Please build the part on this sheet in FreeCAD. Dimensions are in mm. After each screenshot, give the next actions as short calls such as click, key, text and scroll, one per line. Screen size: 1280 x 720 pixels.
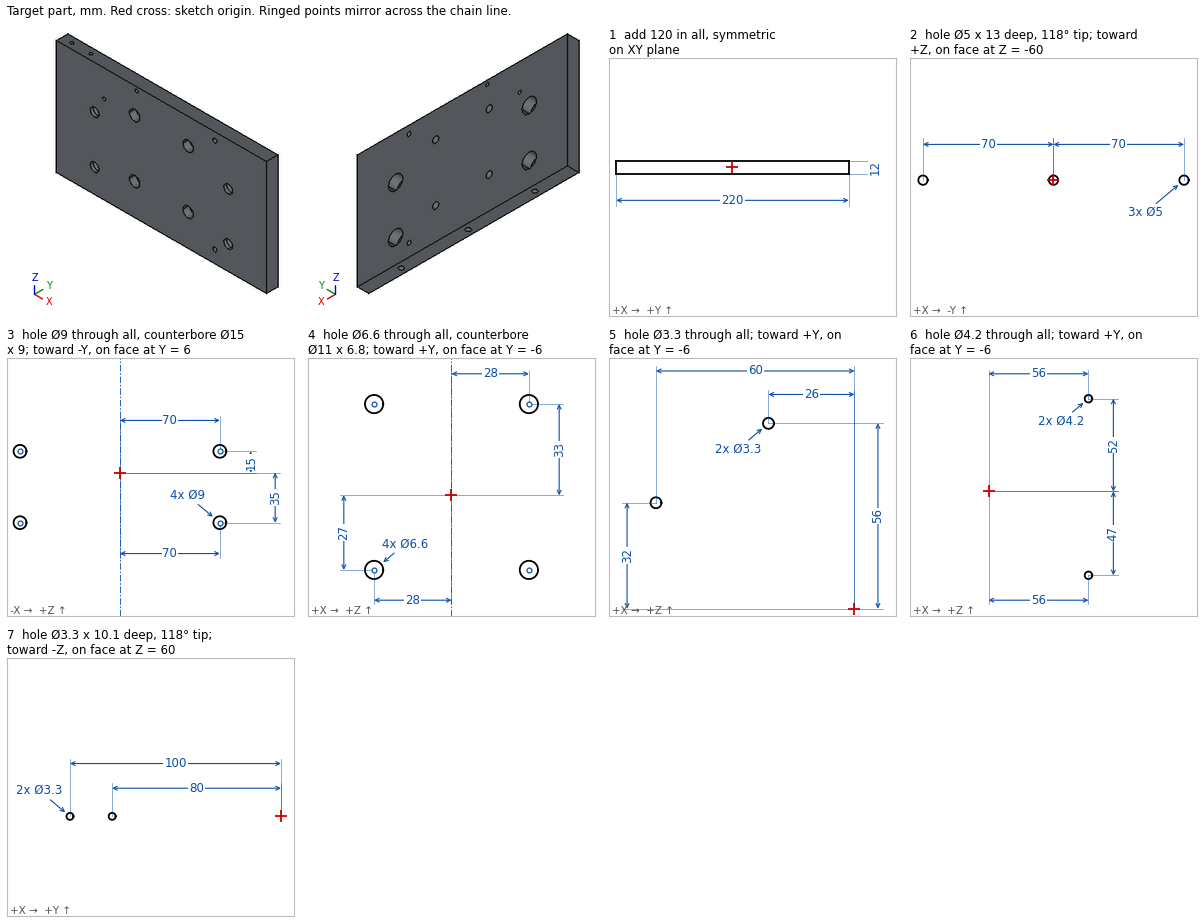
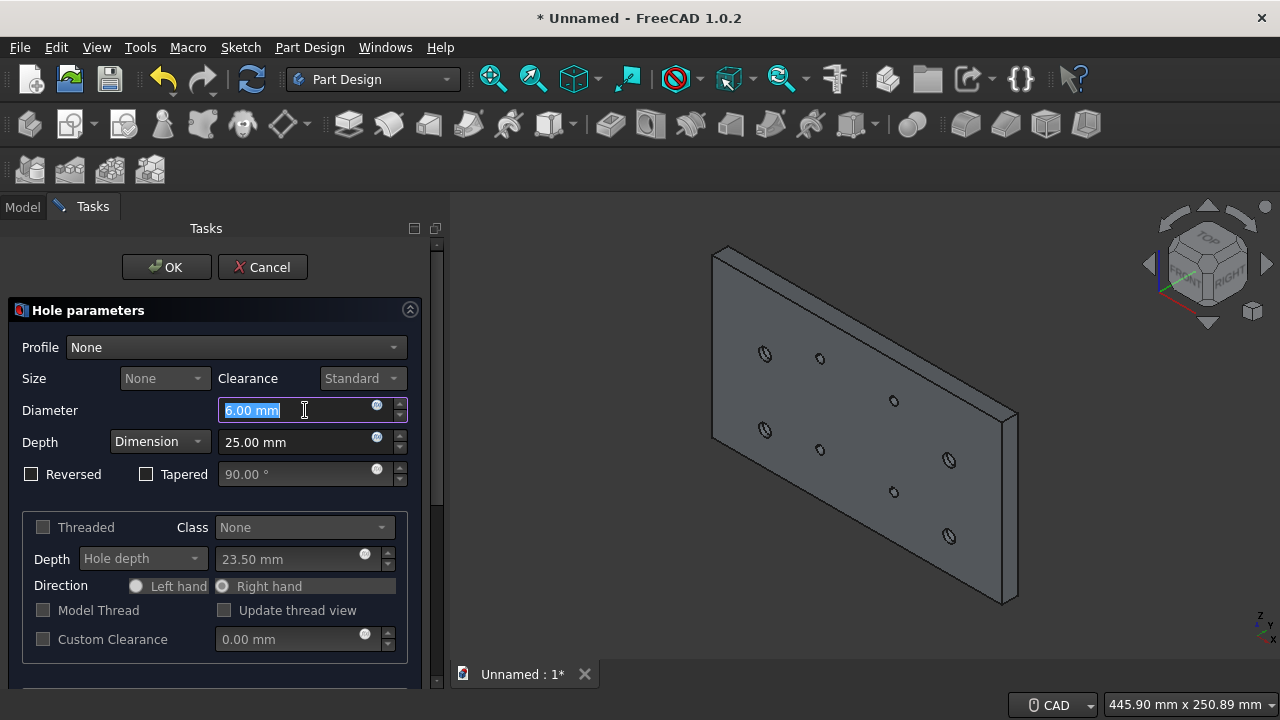
text(6.6)
key(Tab)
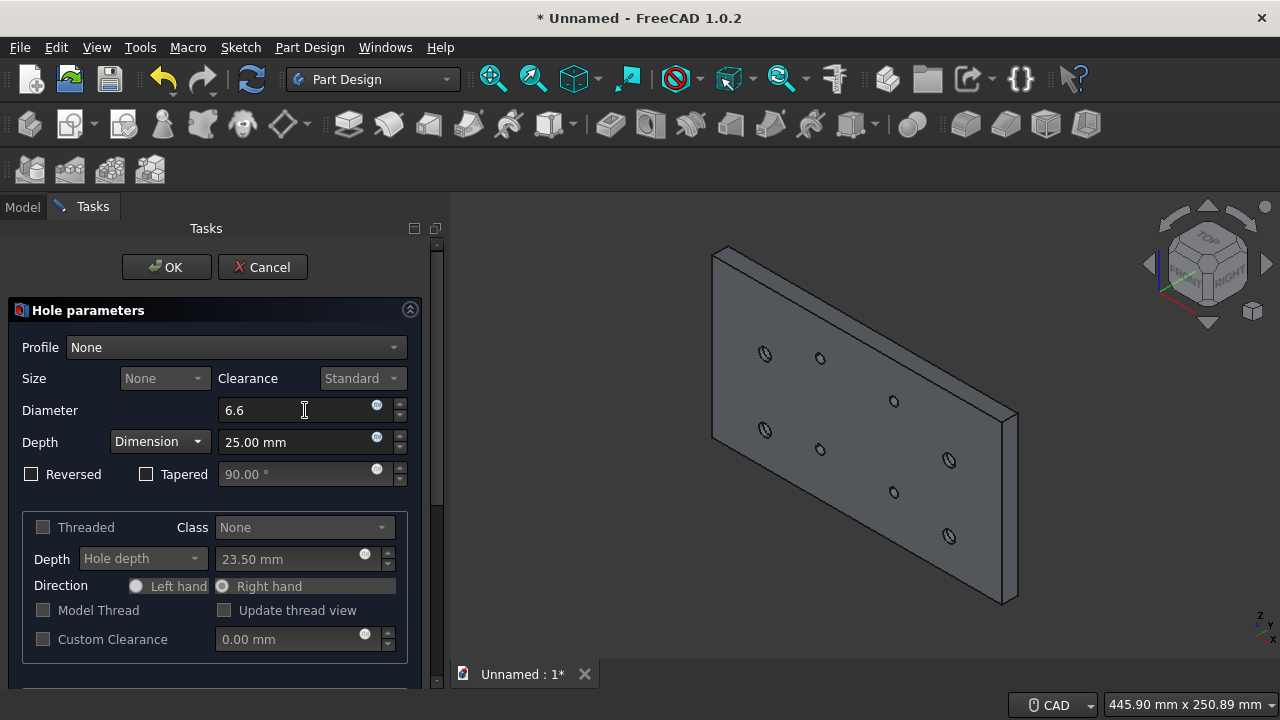
click(161, 442)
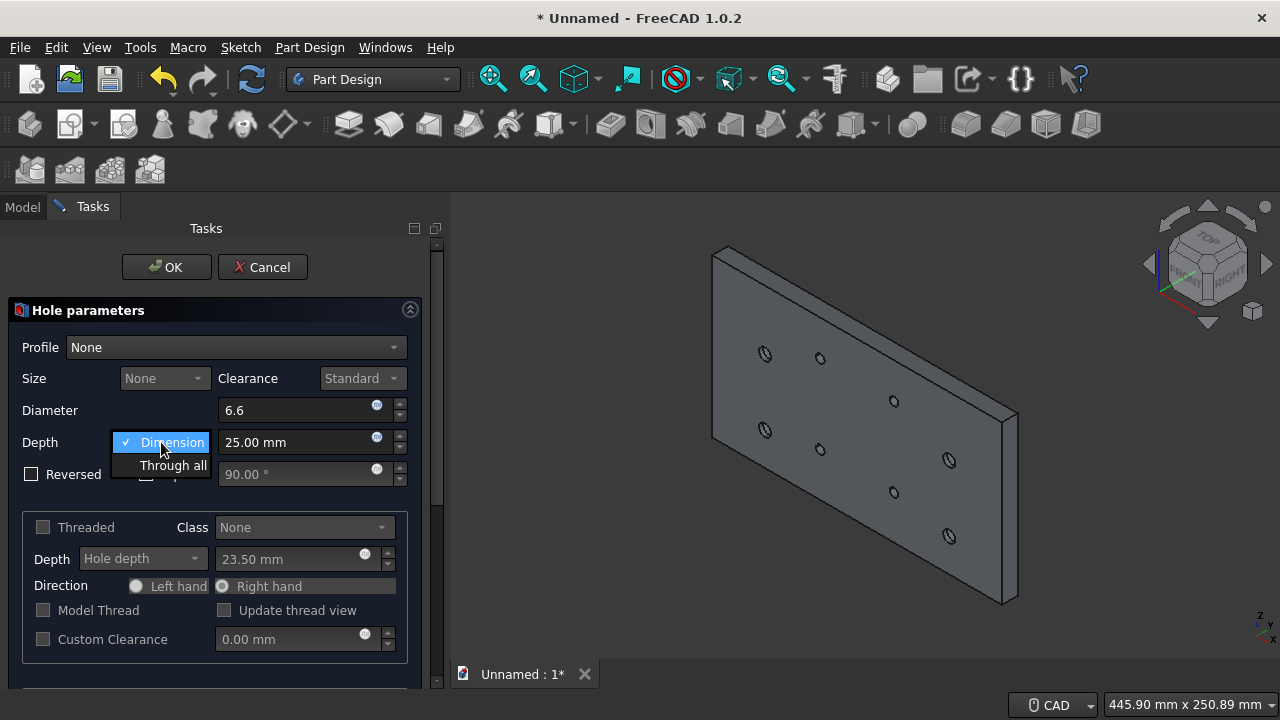
click(160, 466)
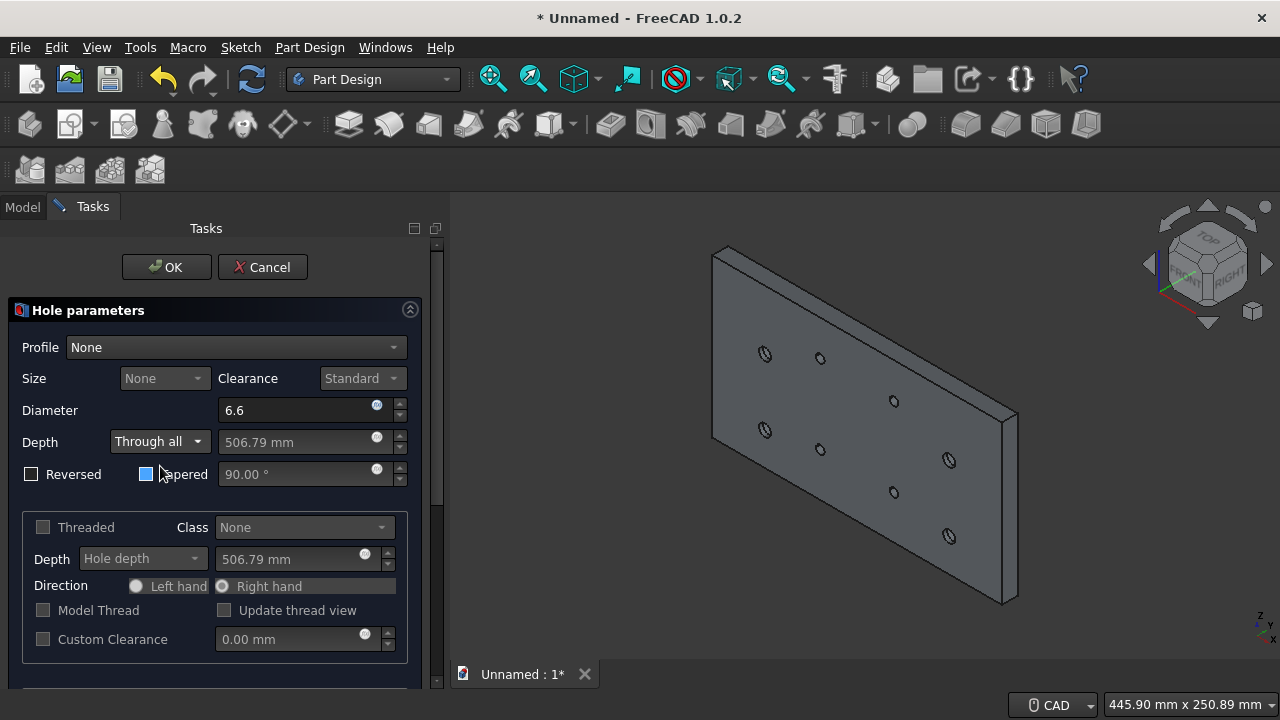
scroll(437, 463, down, 2)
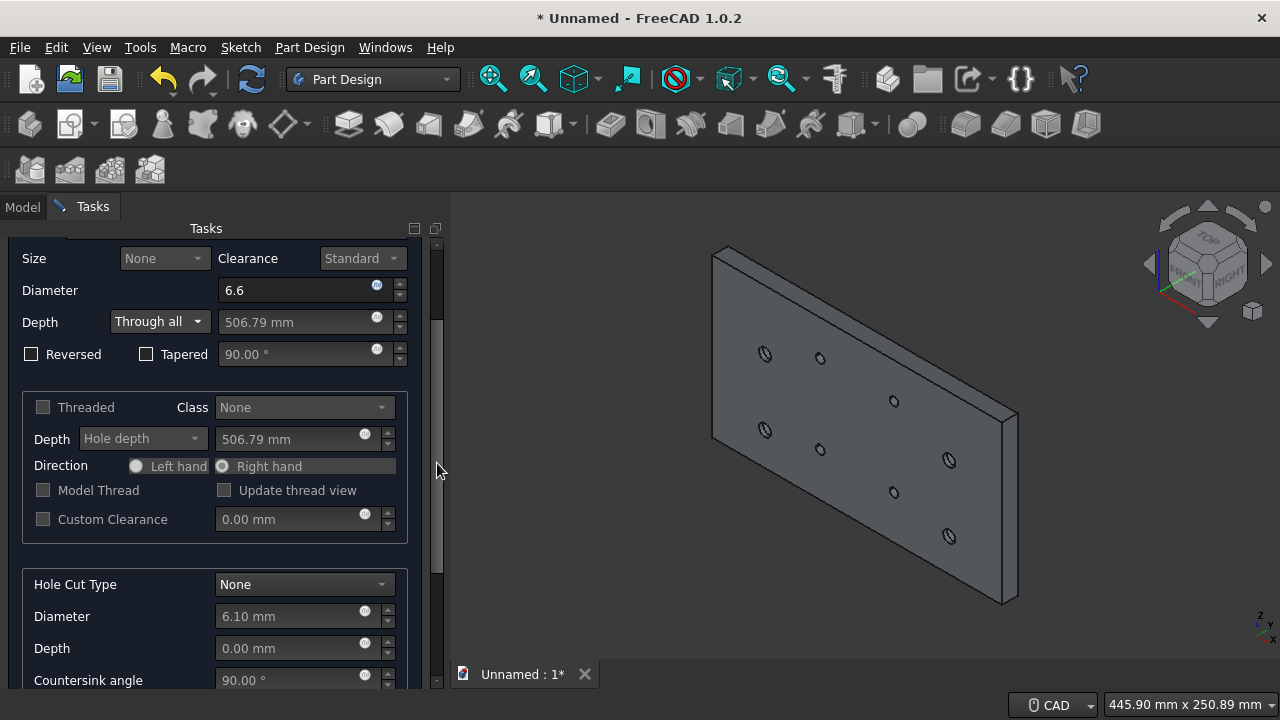
click(306, 584)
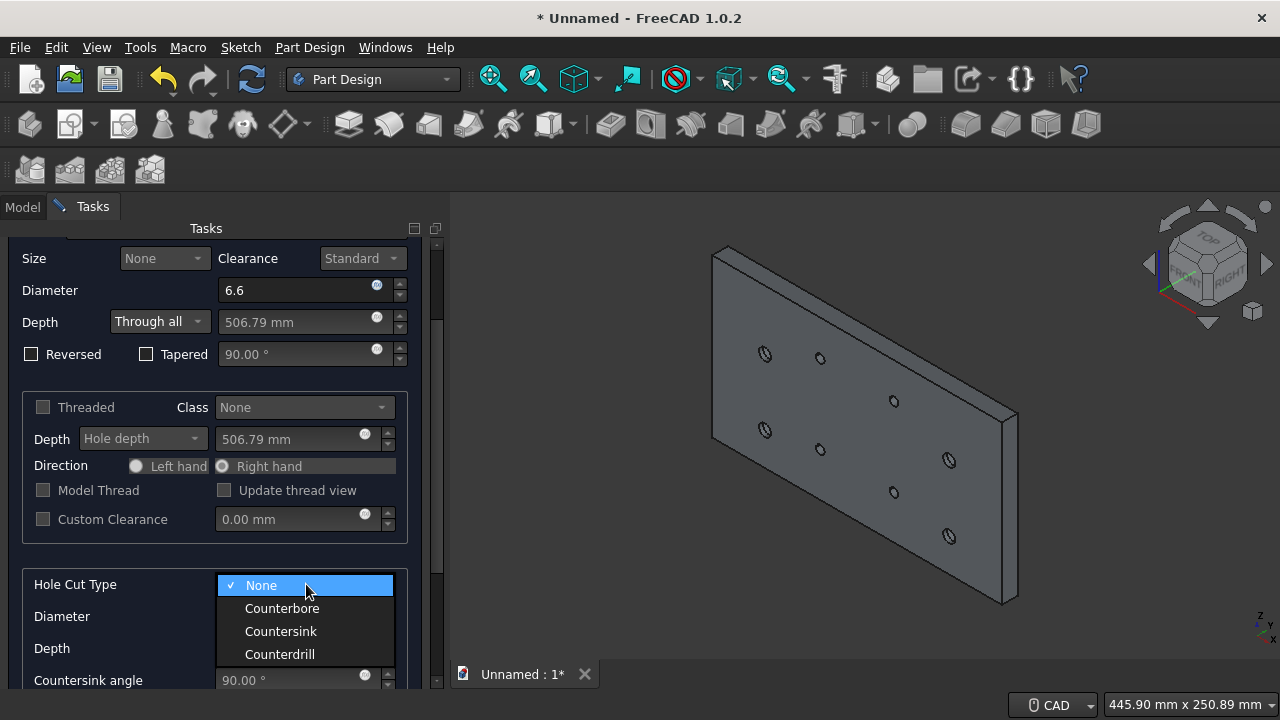
click(304, 608)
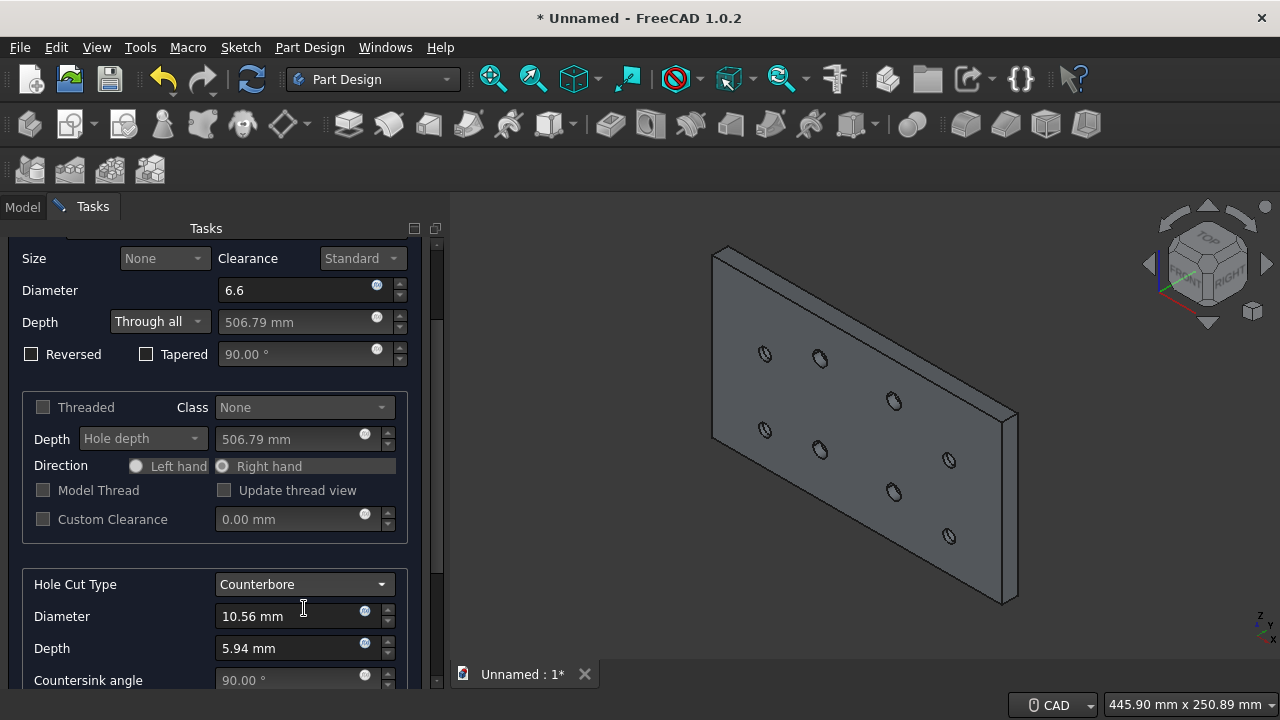
triple_click(298, 616)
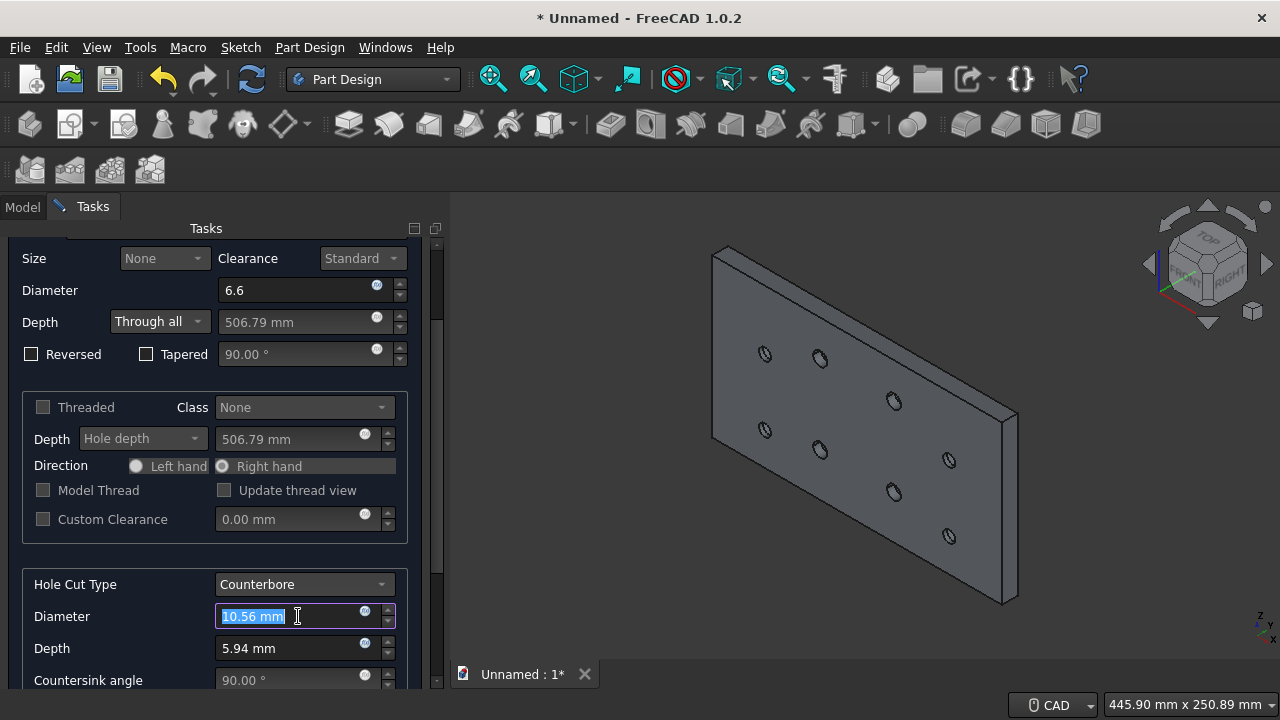
text(11)
key(Tab)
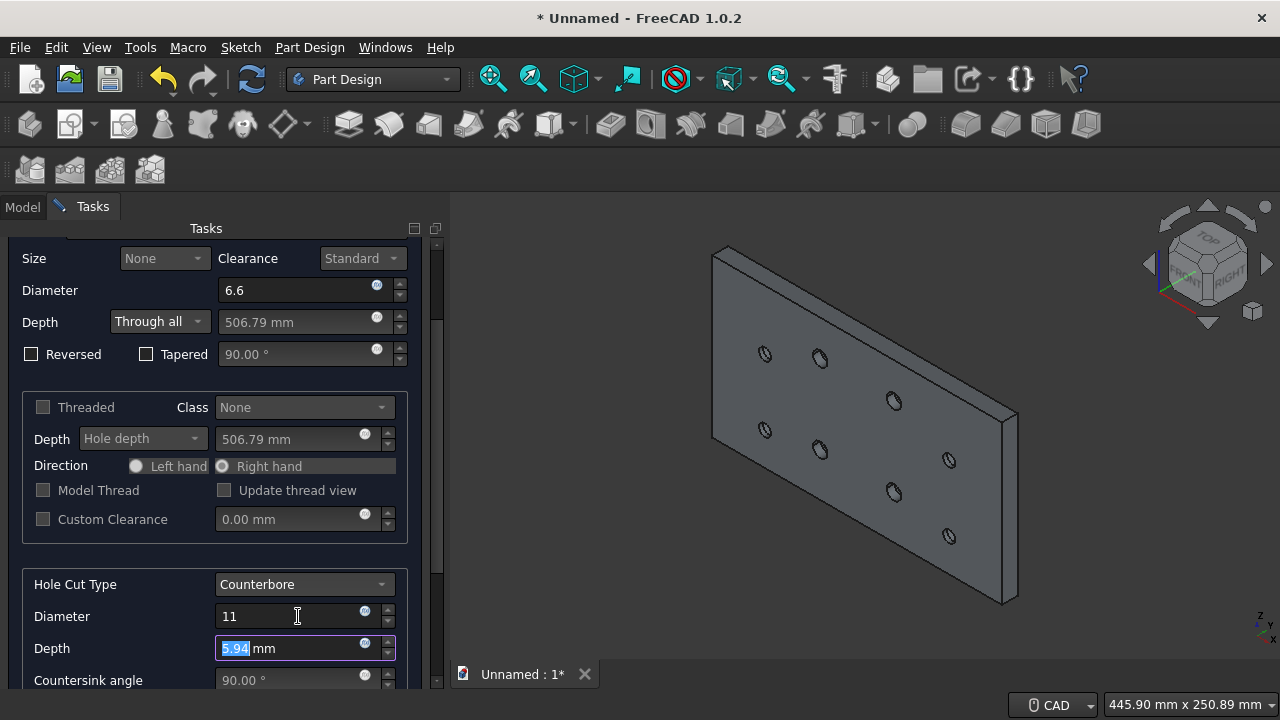
text(6.8)
key(Tab)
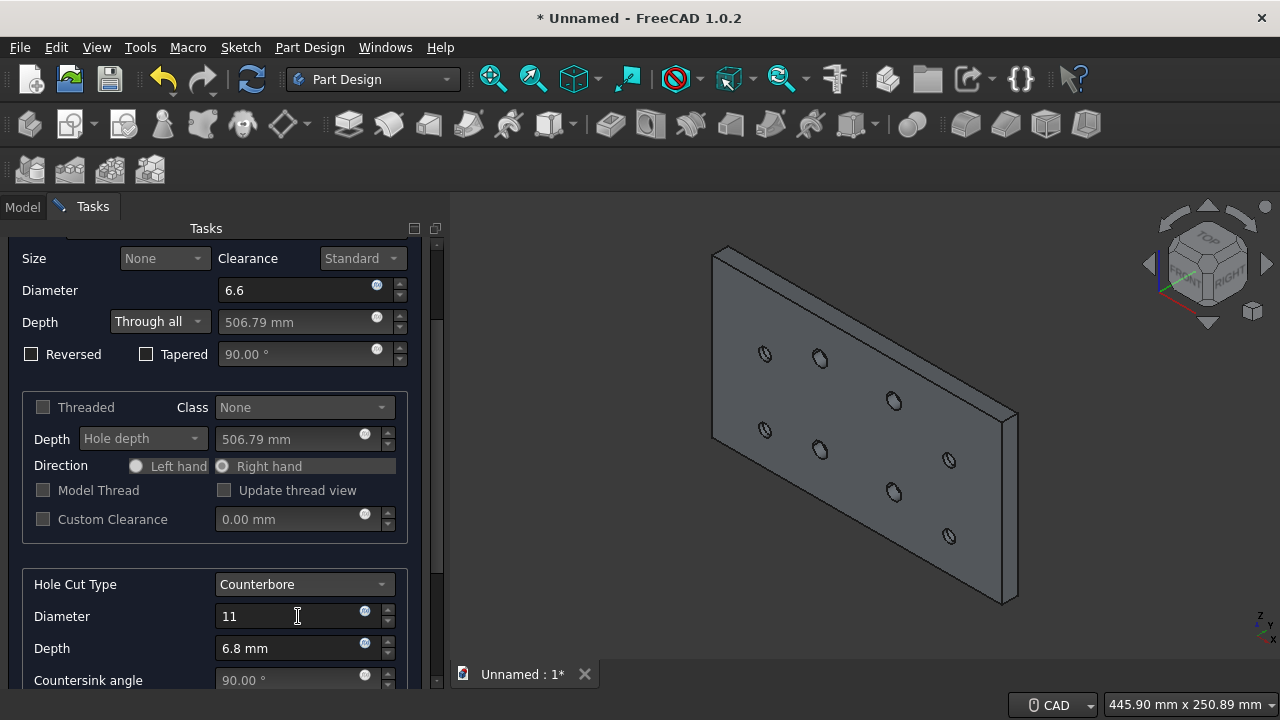
scroll(437, 463, up, 3)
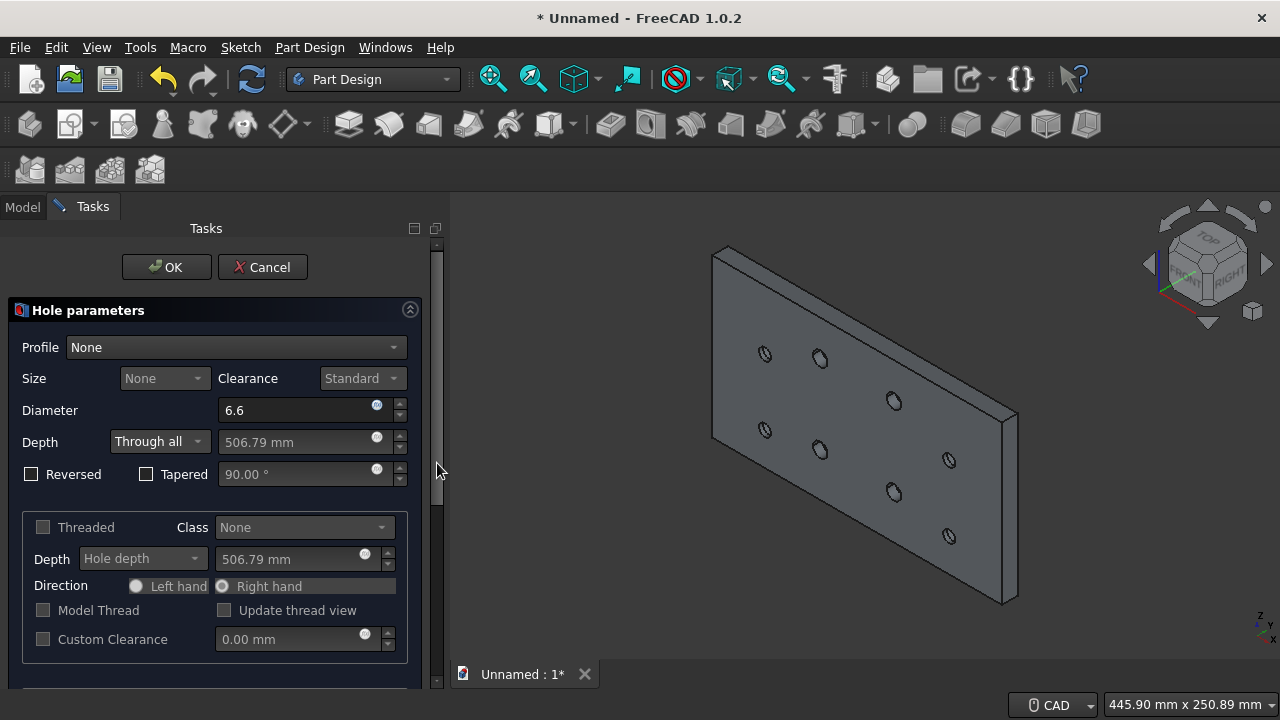
click(167, 267)